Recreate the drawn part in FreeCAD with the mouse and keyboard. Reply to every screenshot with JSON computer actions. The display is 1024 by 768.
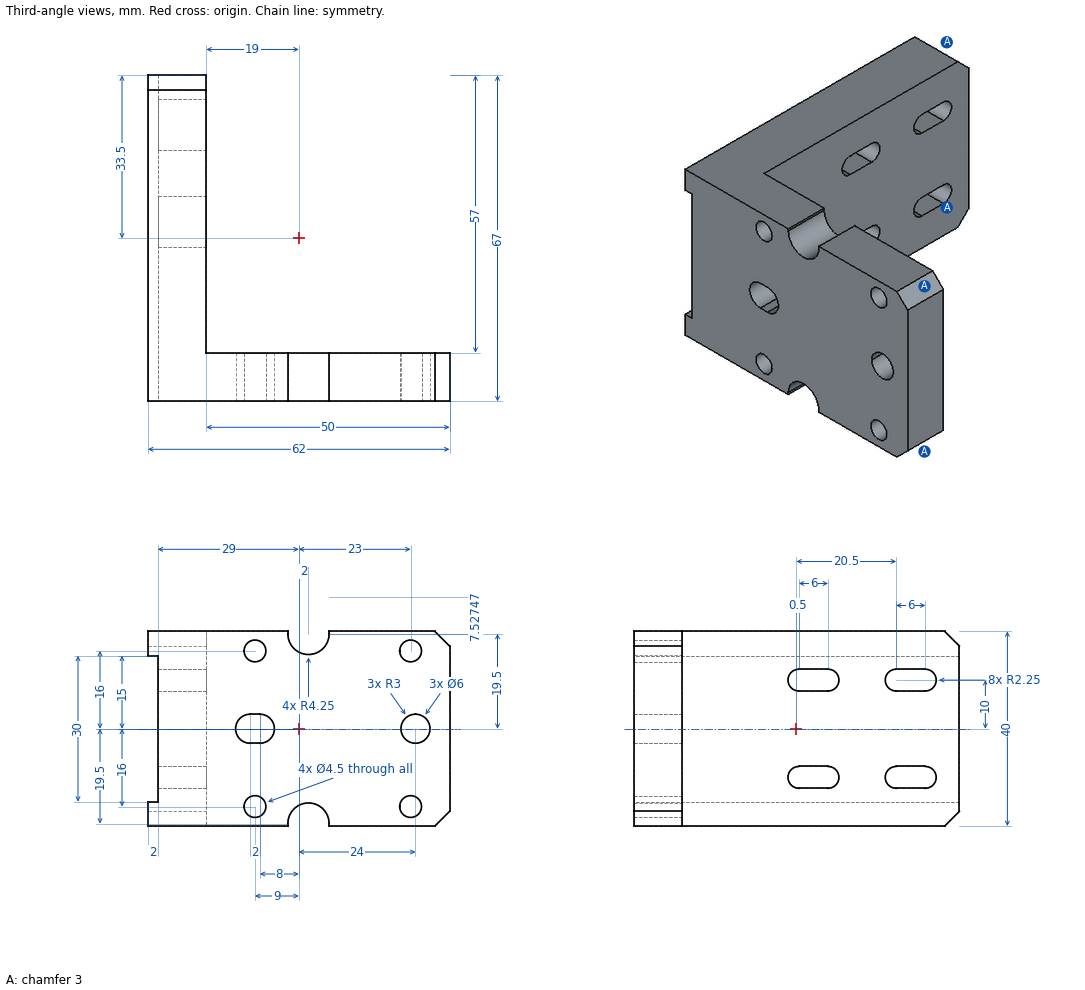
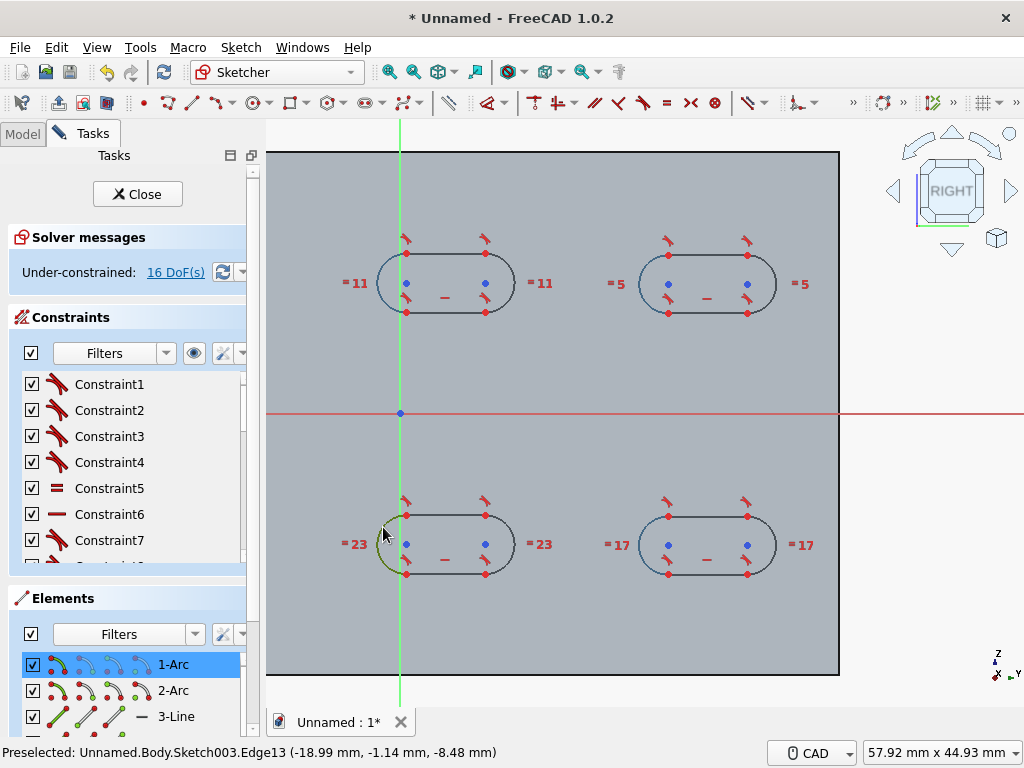
{"action": "left_click", "coordinate": [668, 104]}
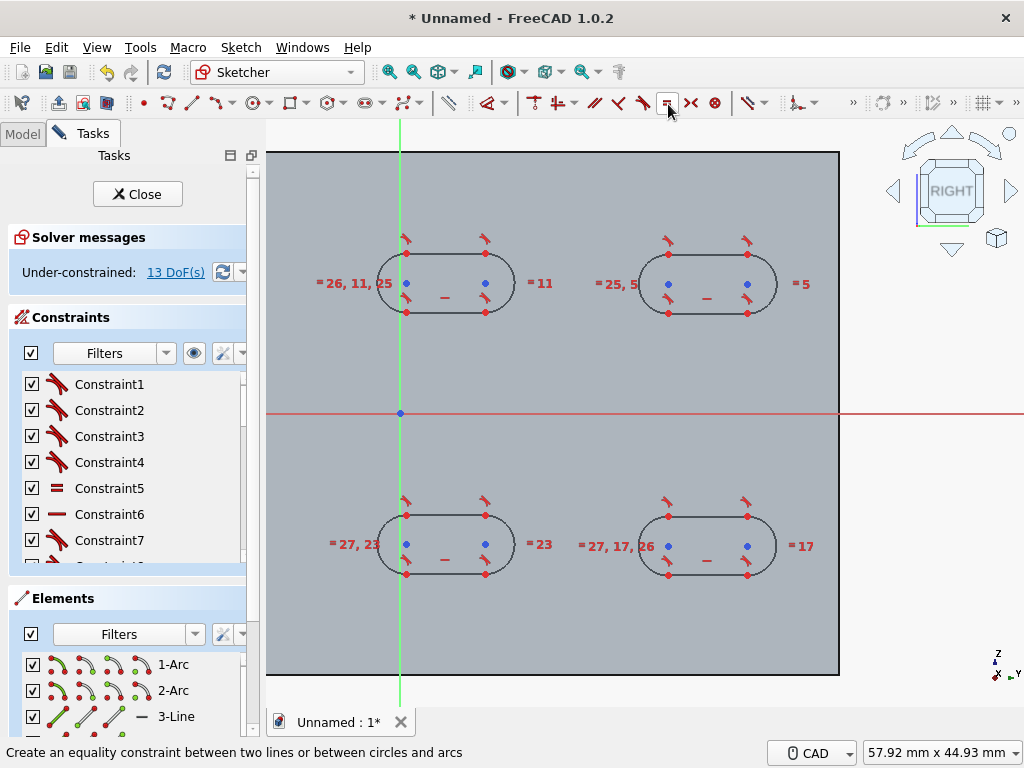
{"action": "left_click", "coordinate": [668, 284]}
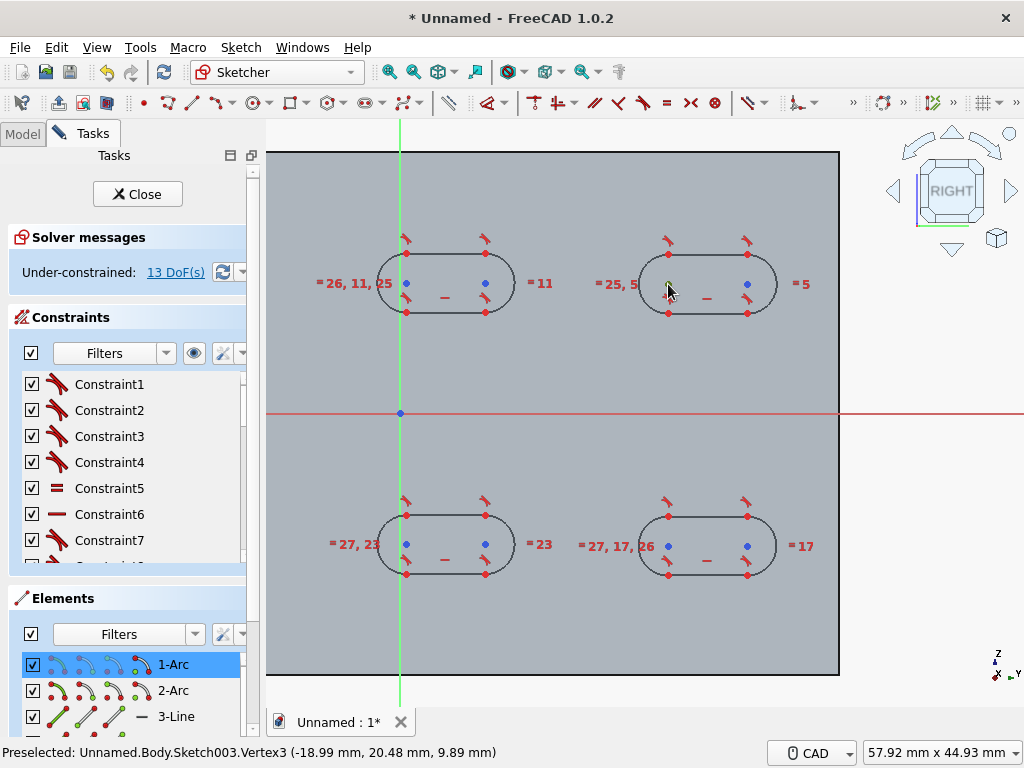
{"action": "left_click", "coordinate": [668, 546]}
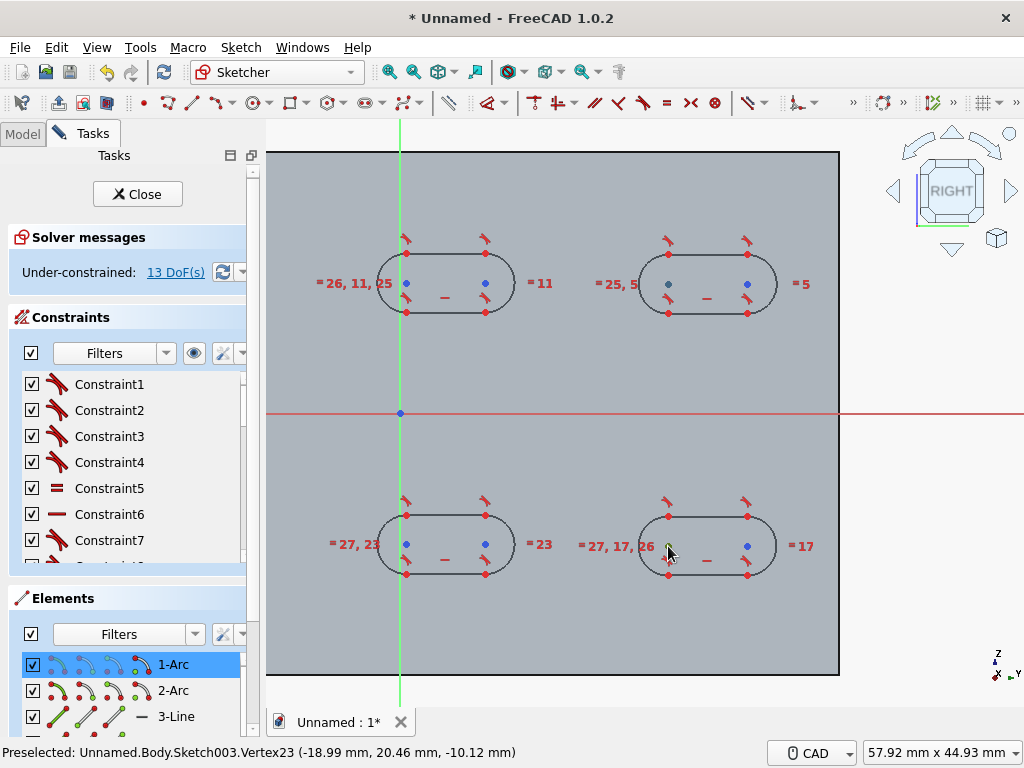
{"action": "left_click", "coordinate": [334, 414]}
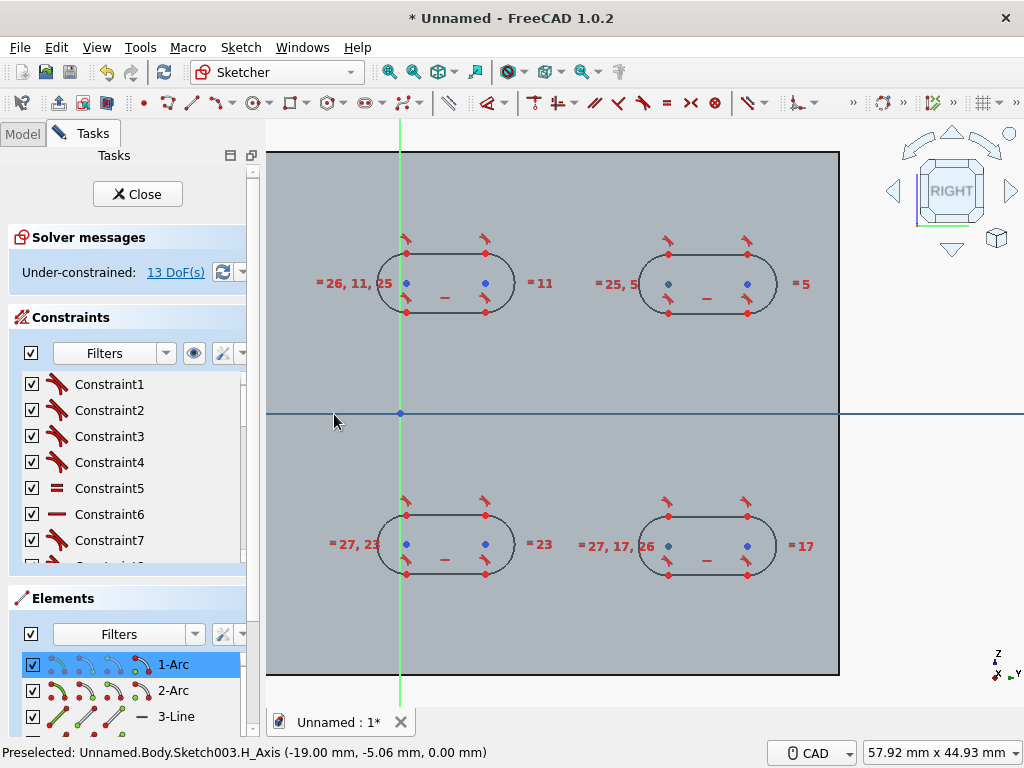
{"action": "left_click", "coordinate": [692, 104]}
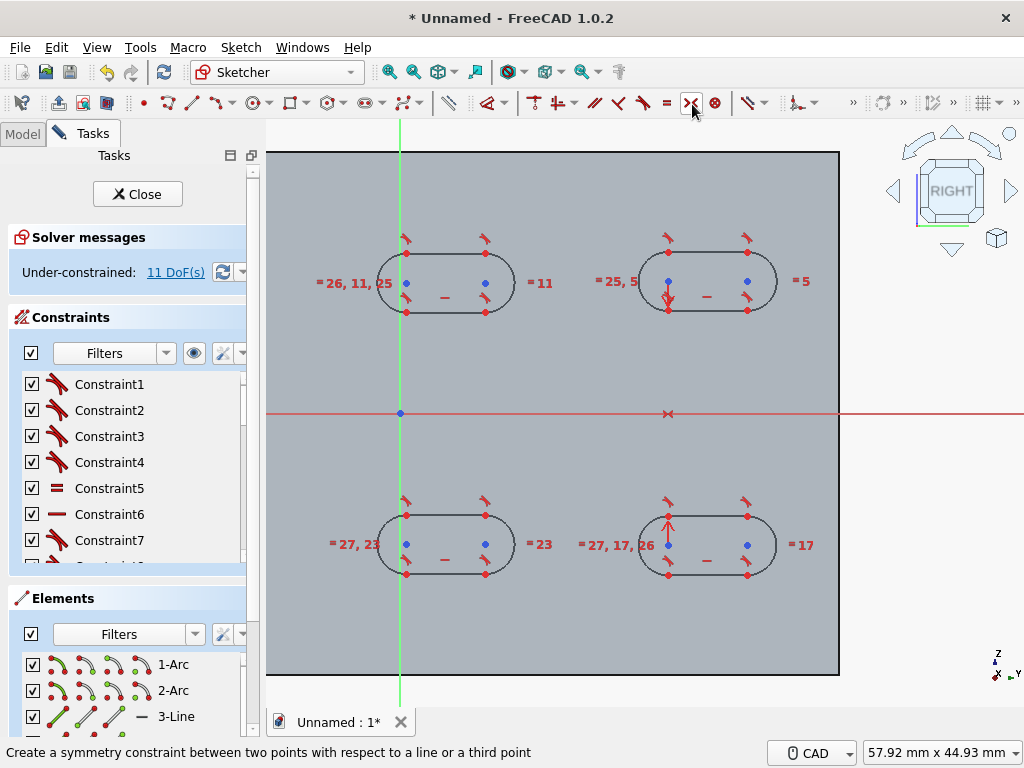
{"action": "left_click", "coordinate": [407, 283]}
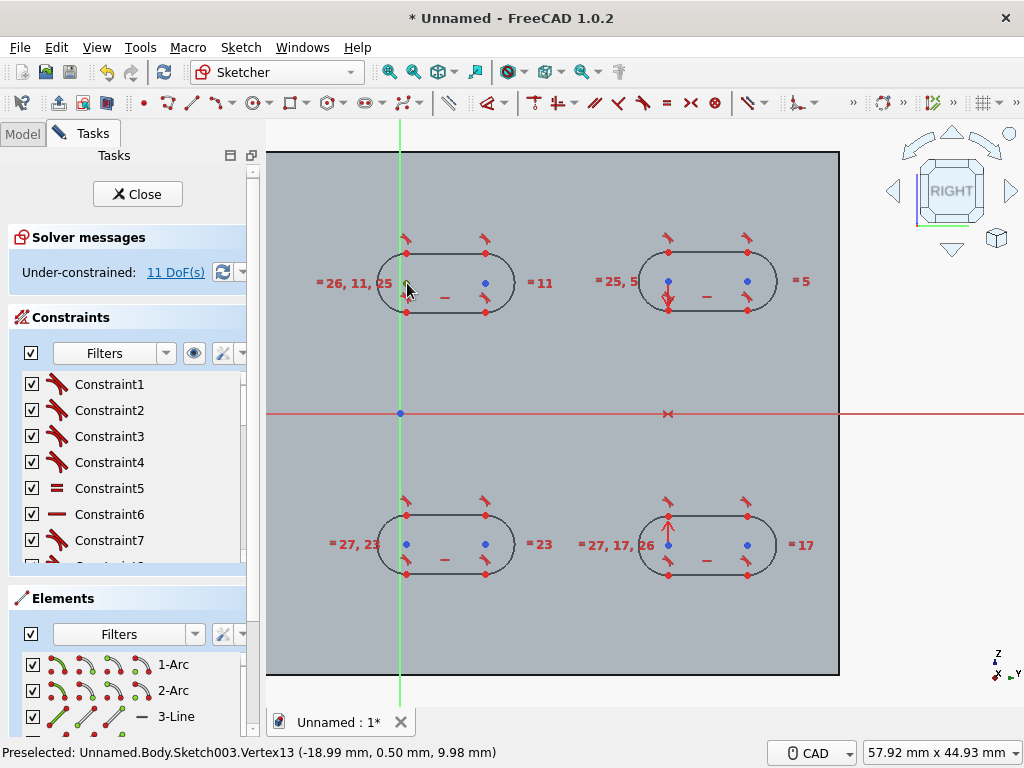
{"action": "left_click", "coordinate": [407, 545]}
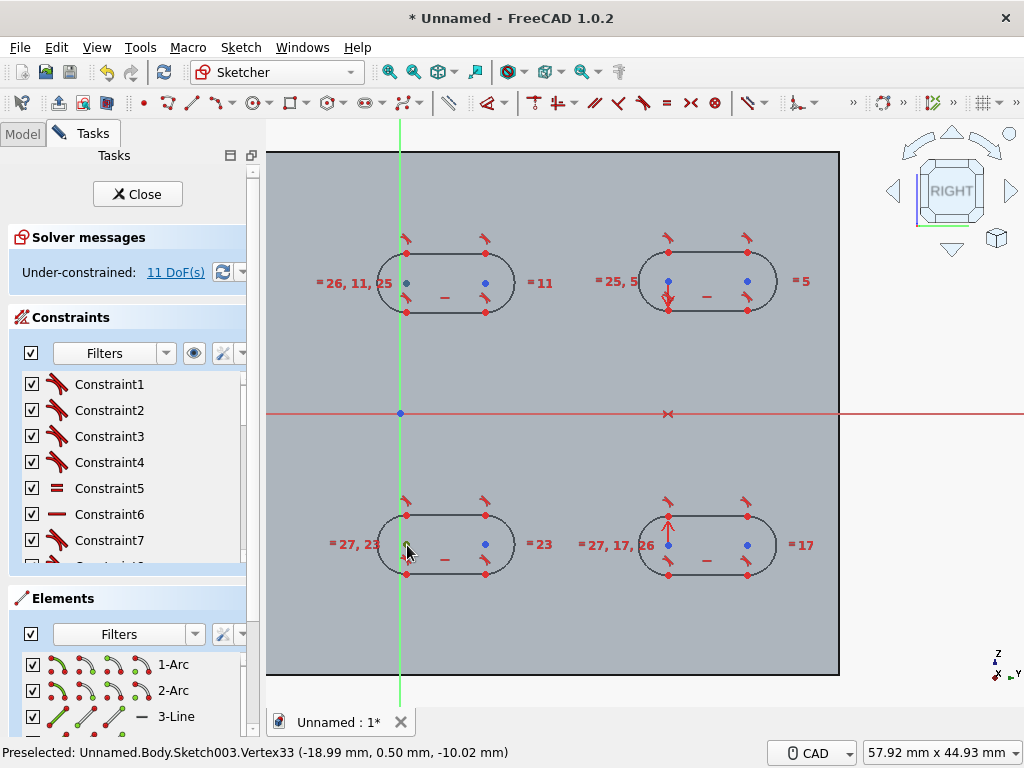
{"action": "left_click", "coordinate": [334, 414]}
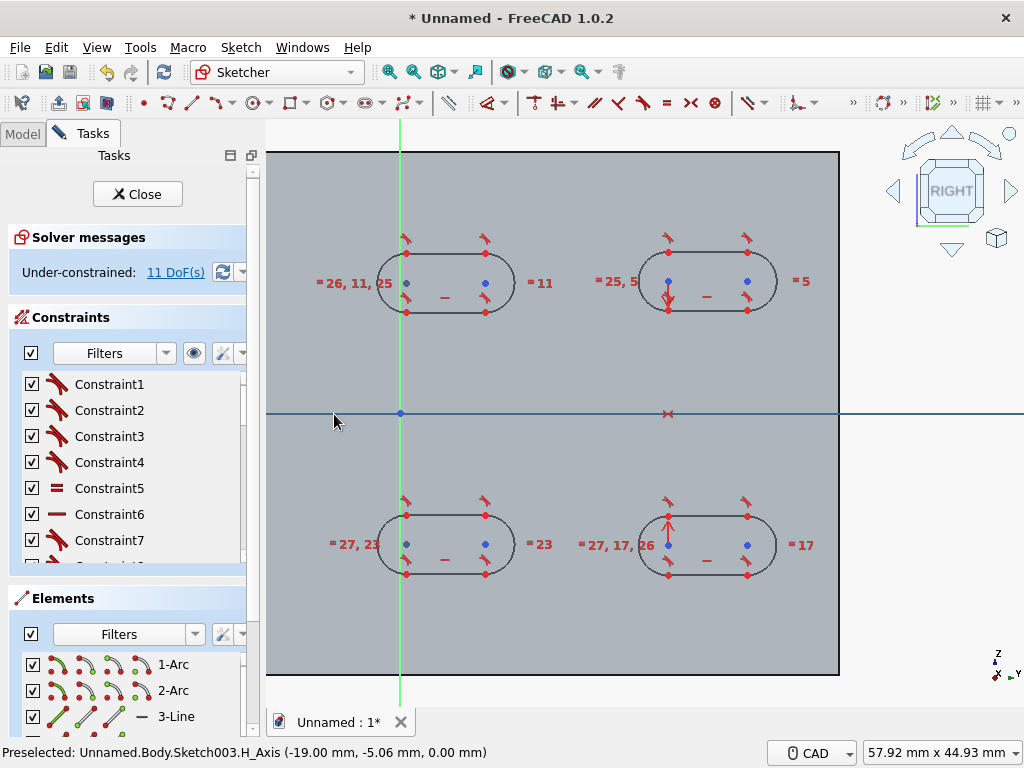
{"action": "left_click", "coordinate": [692, 104]}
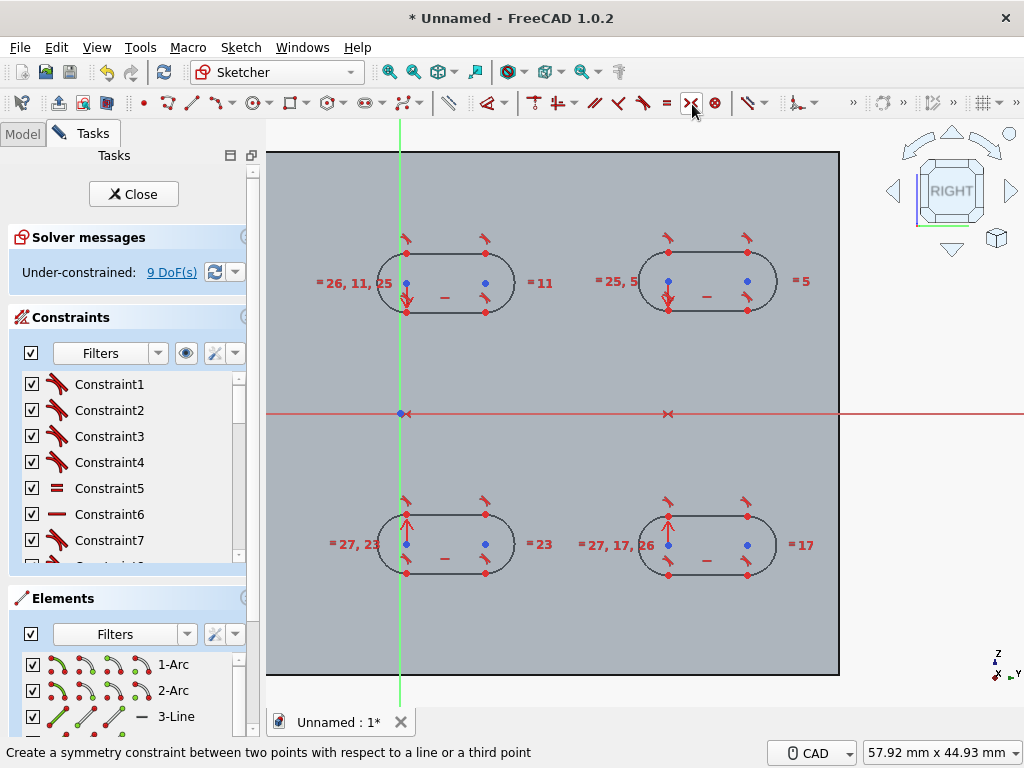
{"action": "left_click", "coordinate": [488, 104]}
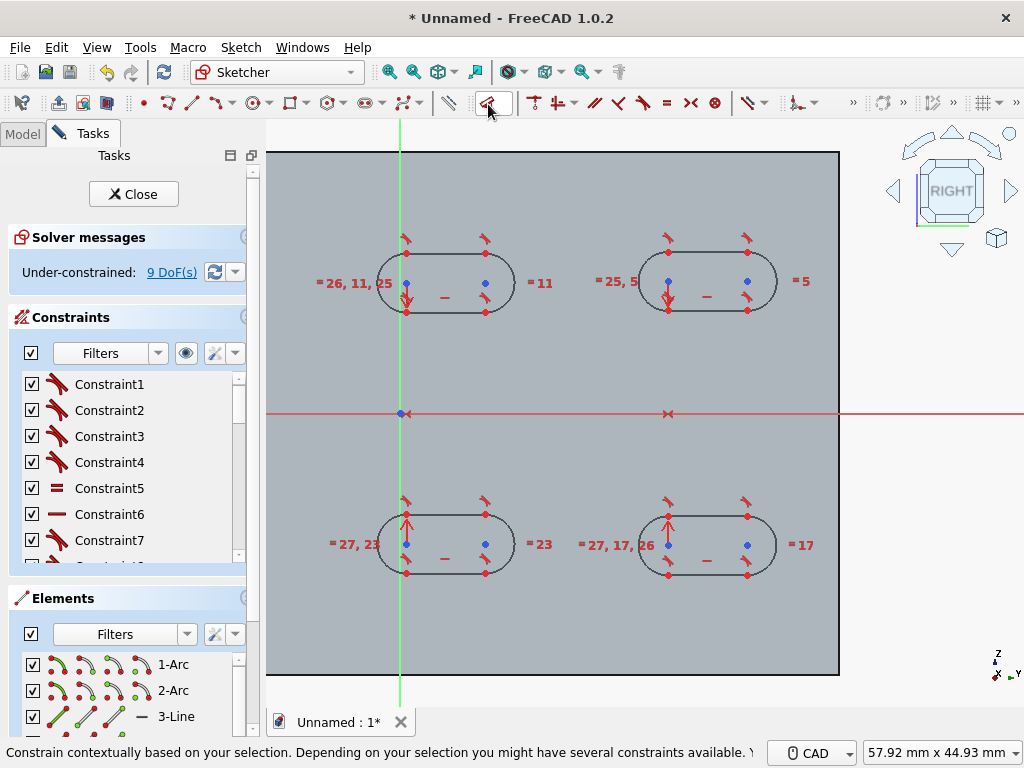
{"action": "scroll", "coordinate": [644, 264], "scroll_direction": "up", "scroll_amount": 2}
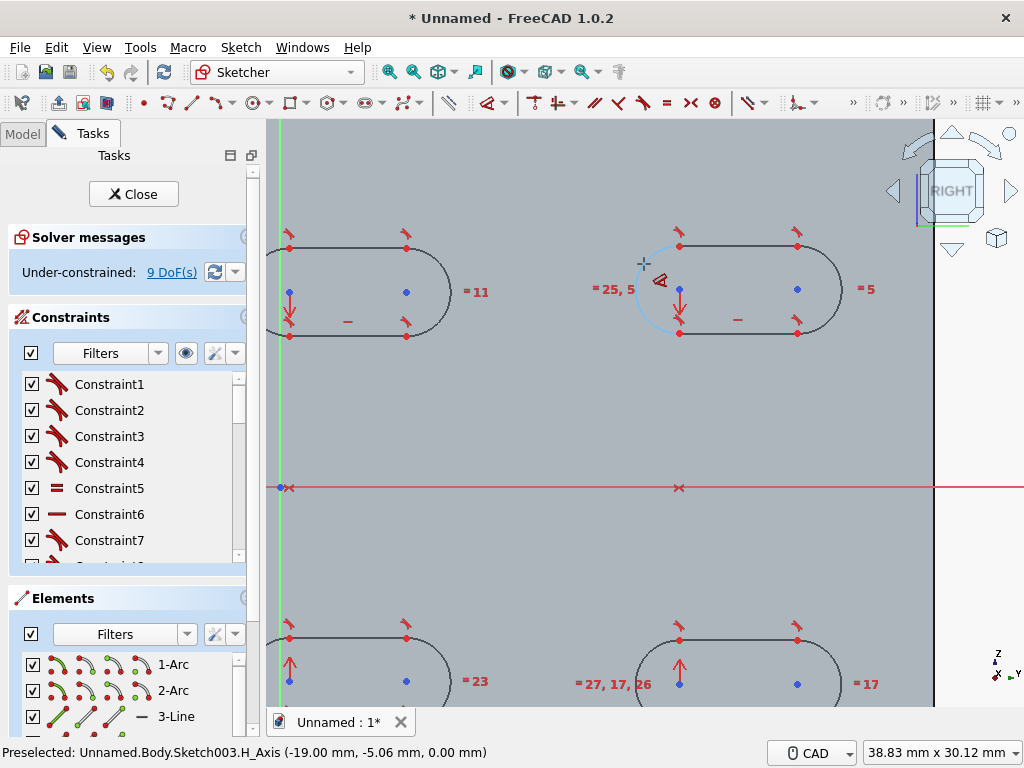
{"action": "left_click", "coordinate": [644, 264]}
{"action": "left_click", "coordinate": [618, 245]}